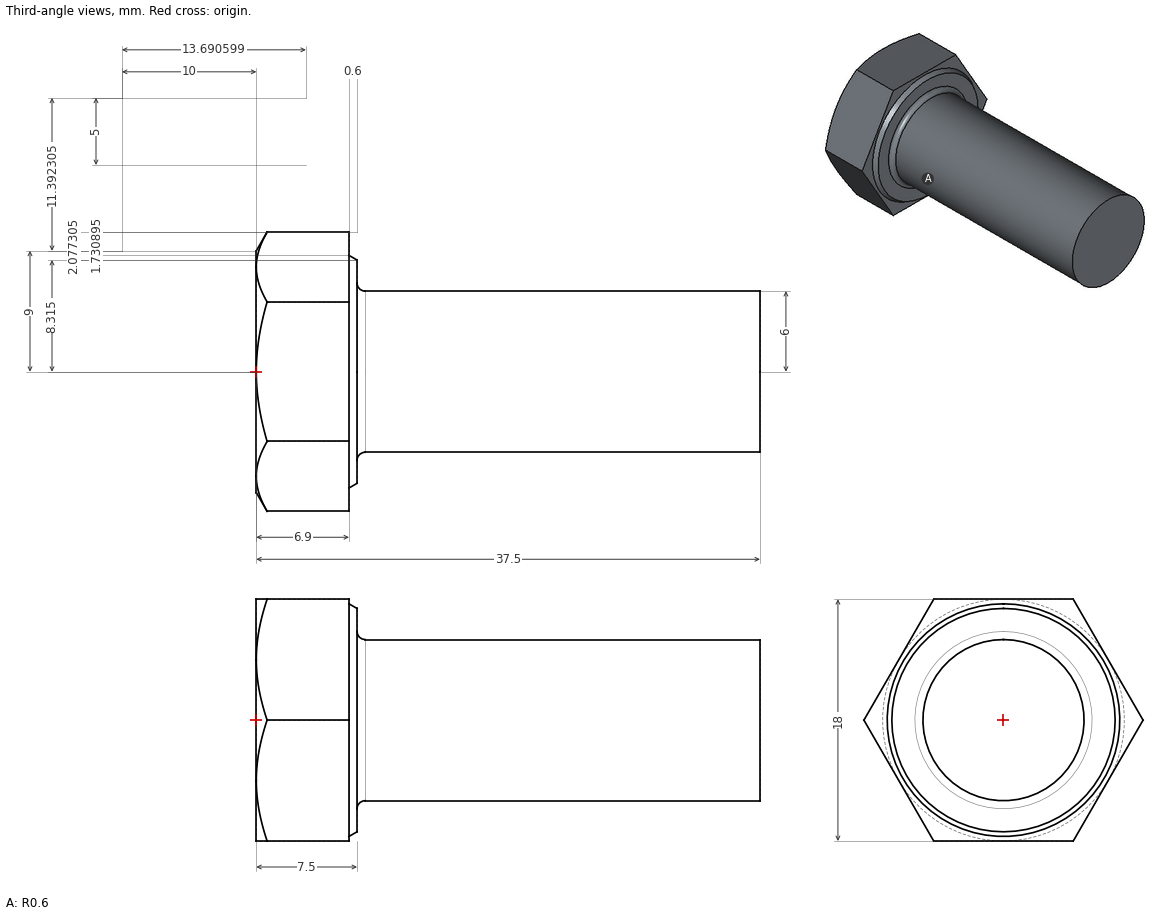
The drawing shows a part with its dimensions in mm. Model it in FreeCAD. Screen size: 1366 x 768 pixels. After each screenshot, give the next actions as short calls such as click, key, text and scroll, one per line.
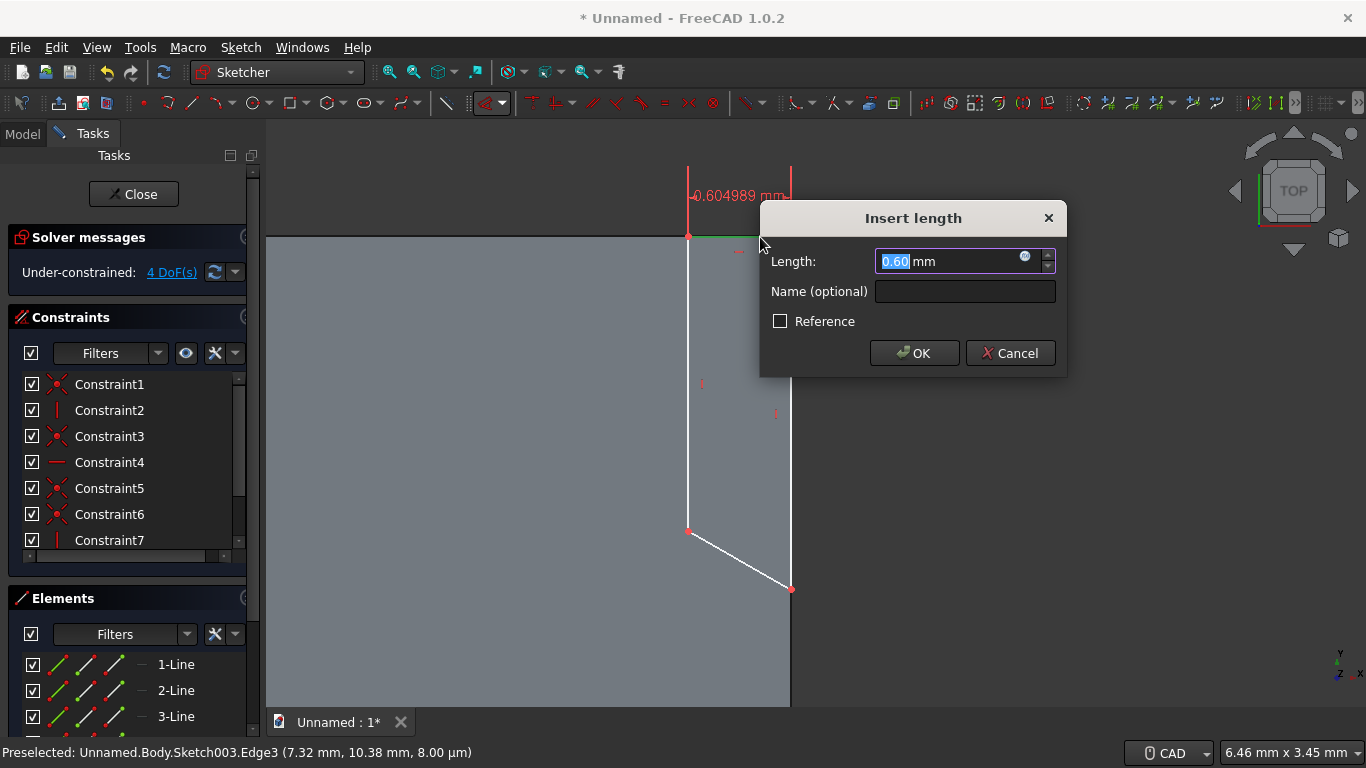
text(0.6)
key(Return)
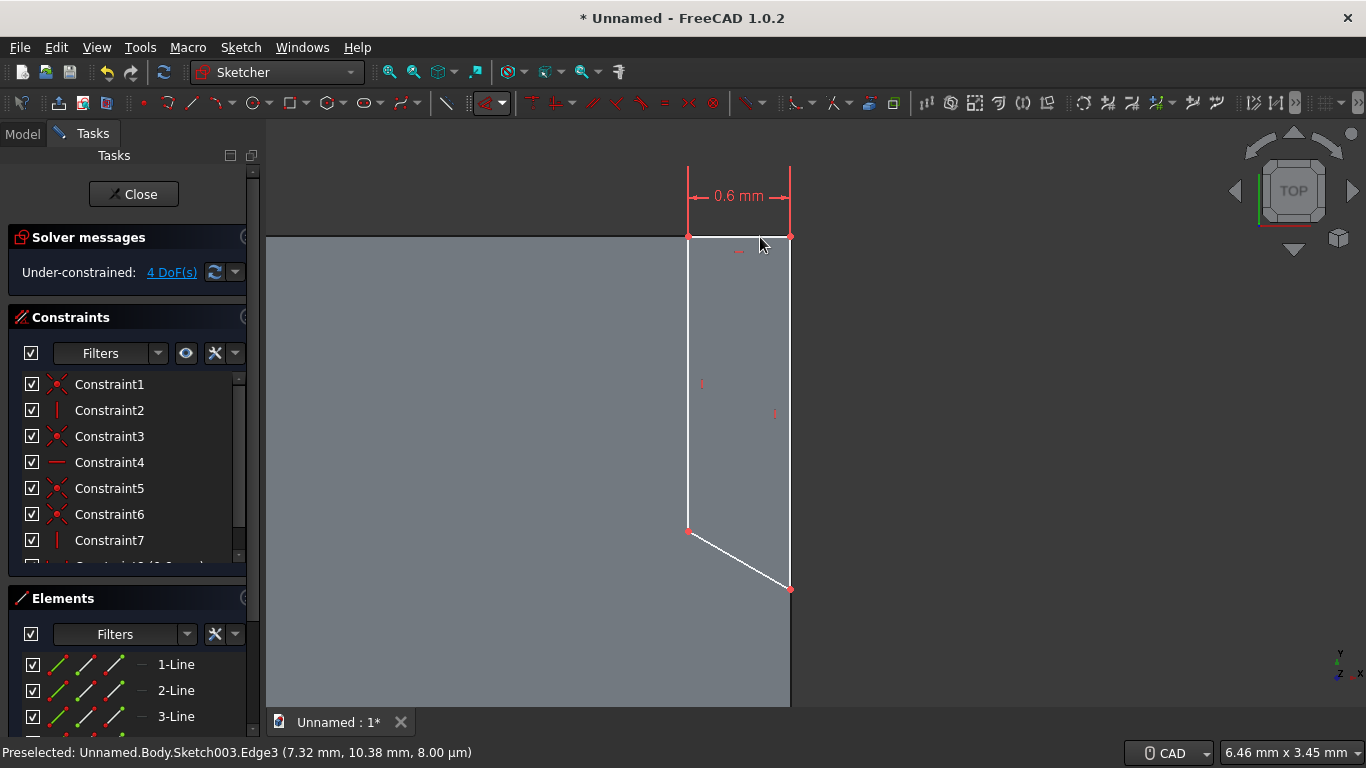
click(688, 531)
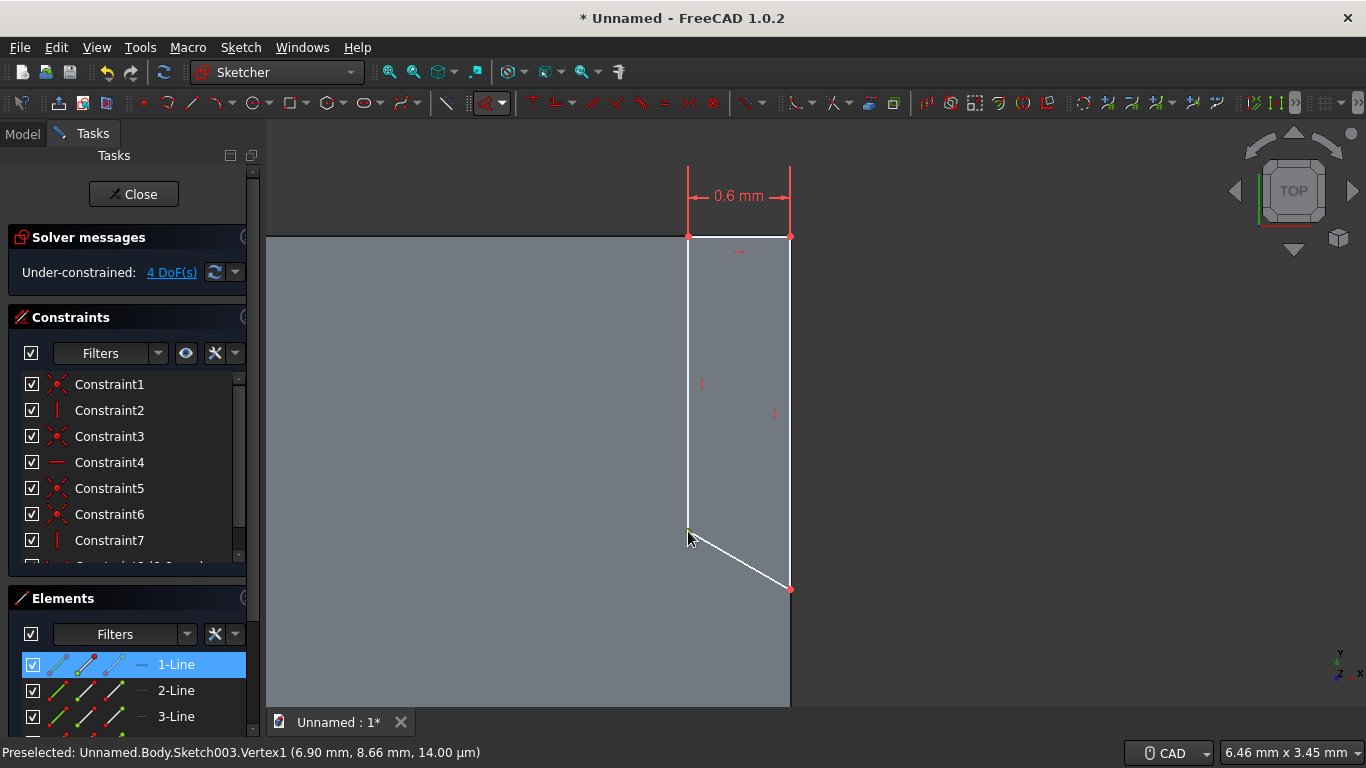
key(l)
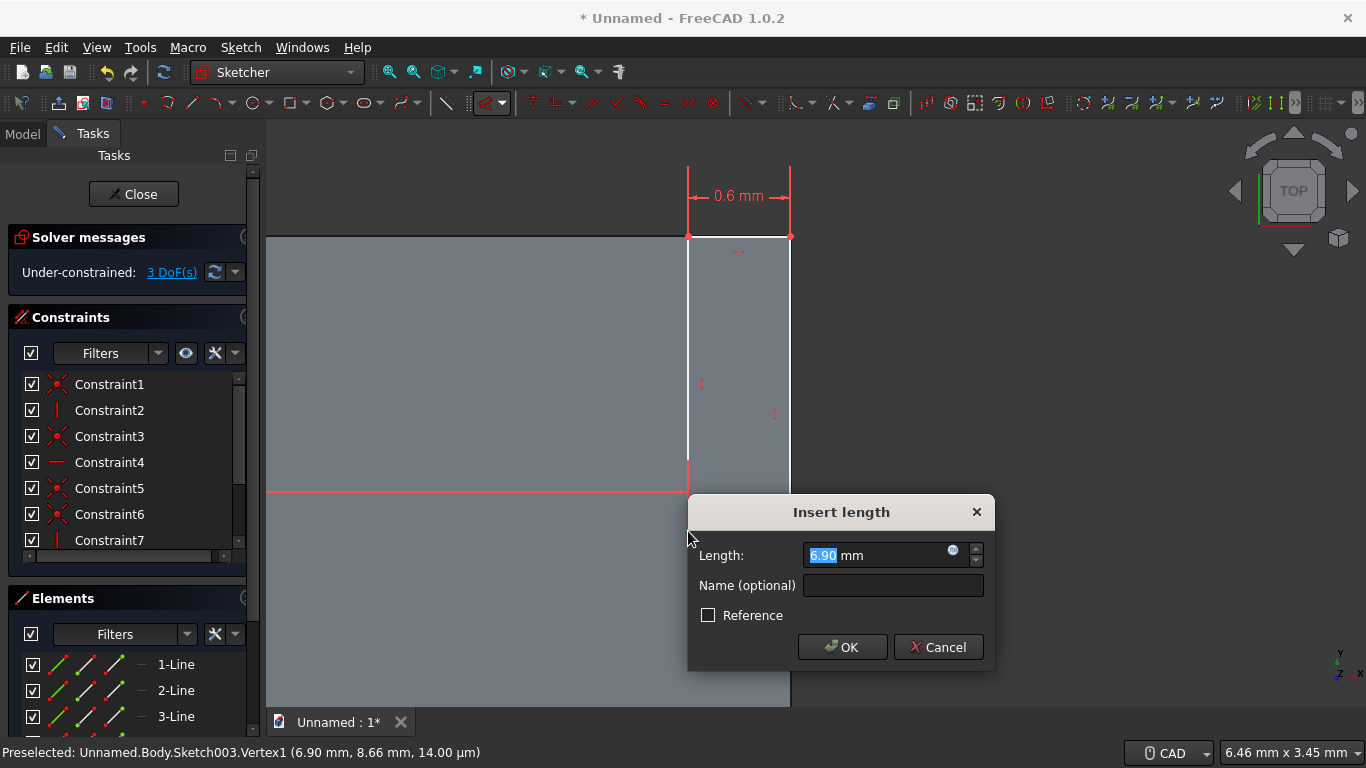
text(6.9)
key(Return)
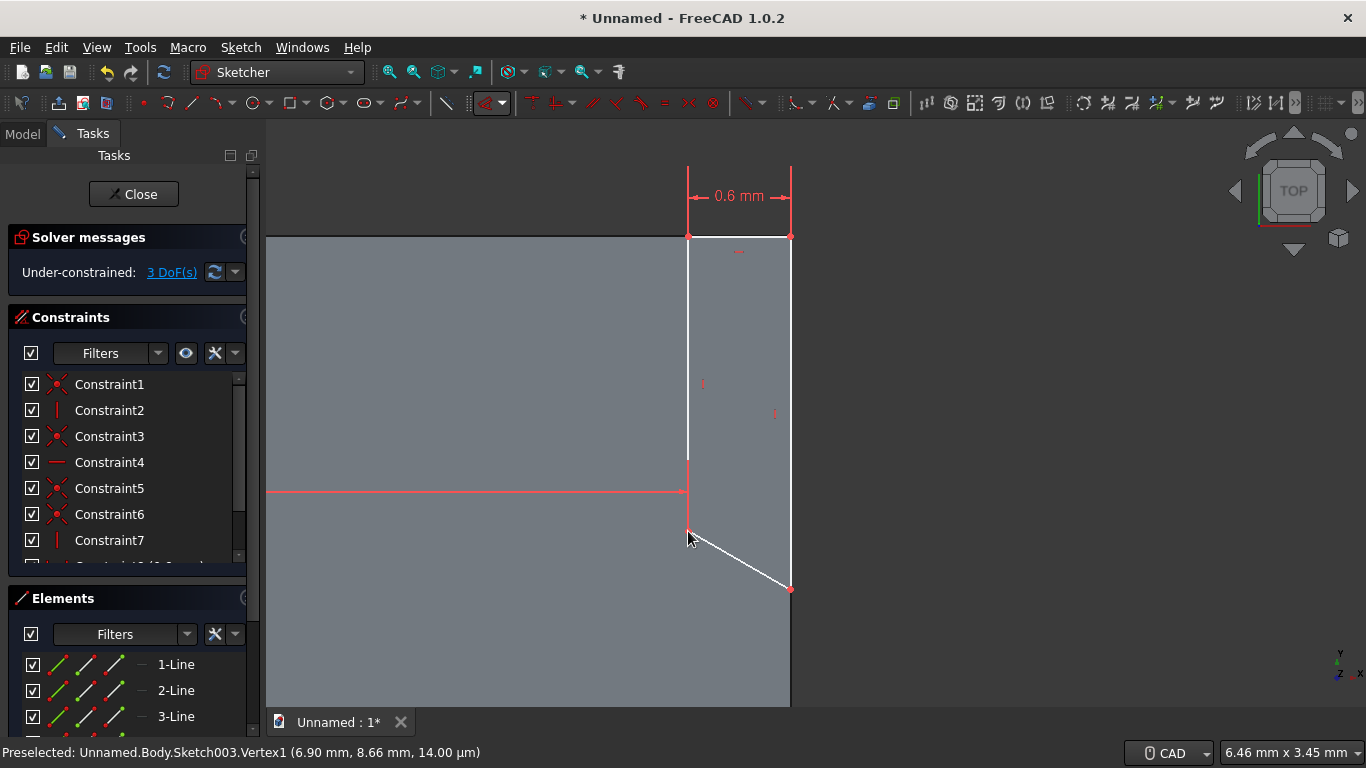
click(791, 590)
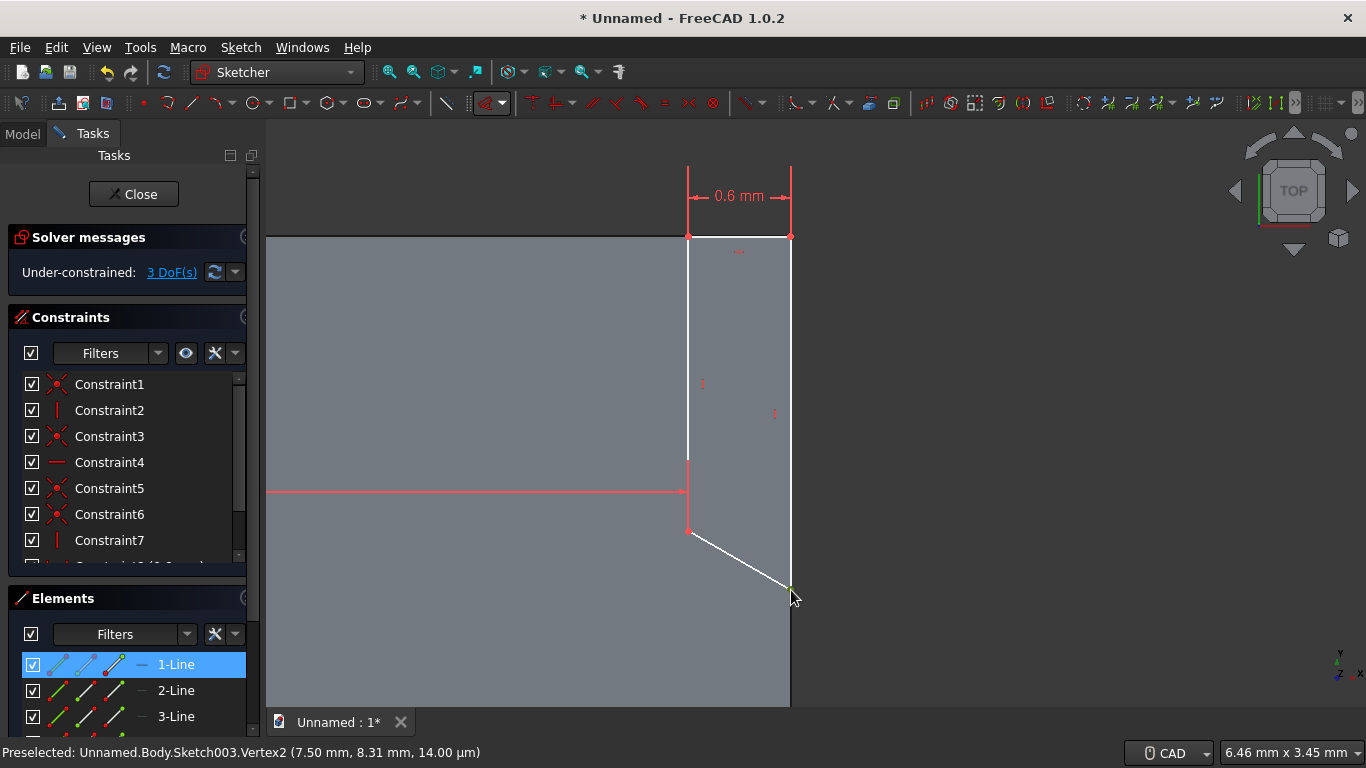
key(i)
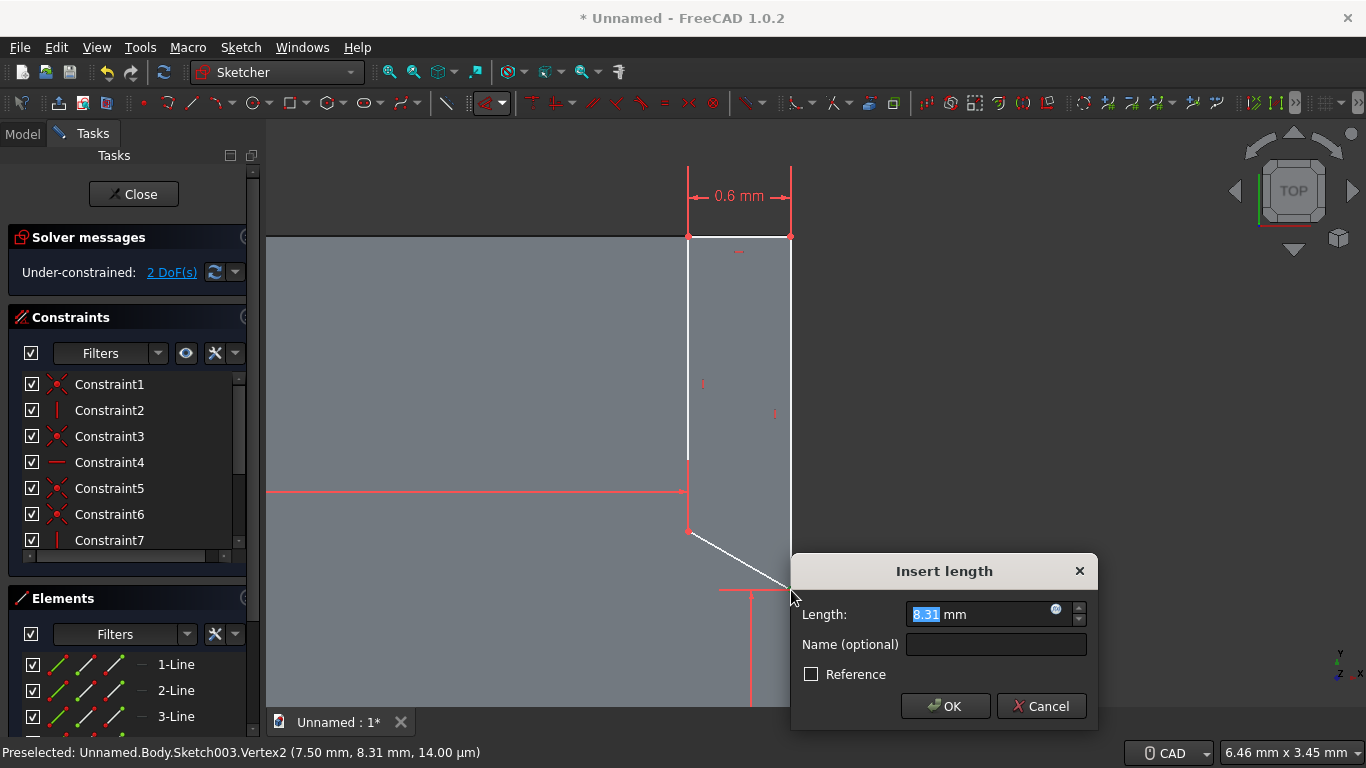
text(8.315)
key(Return)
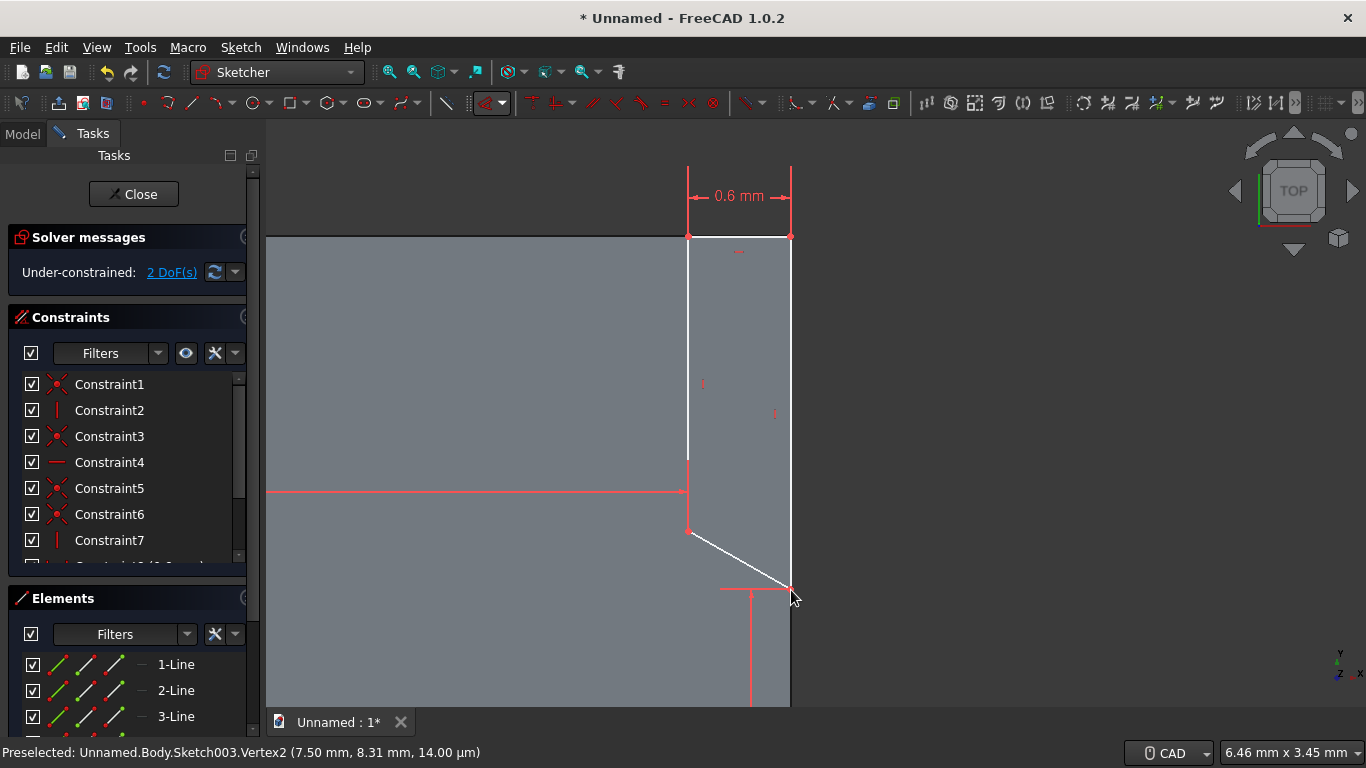
click(791, 484)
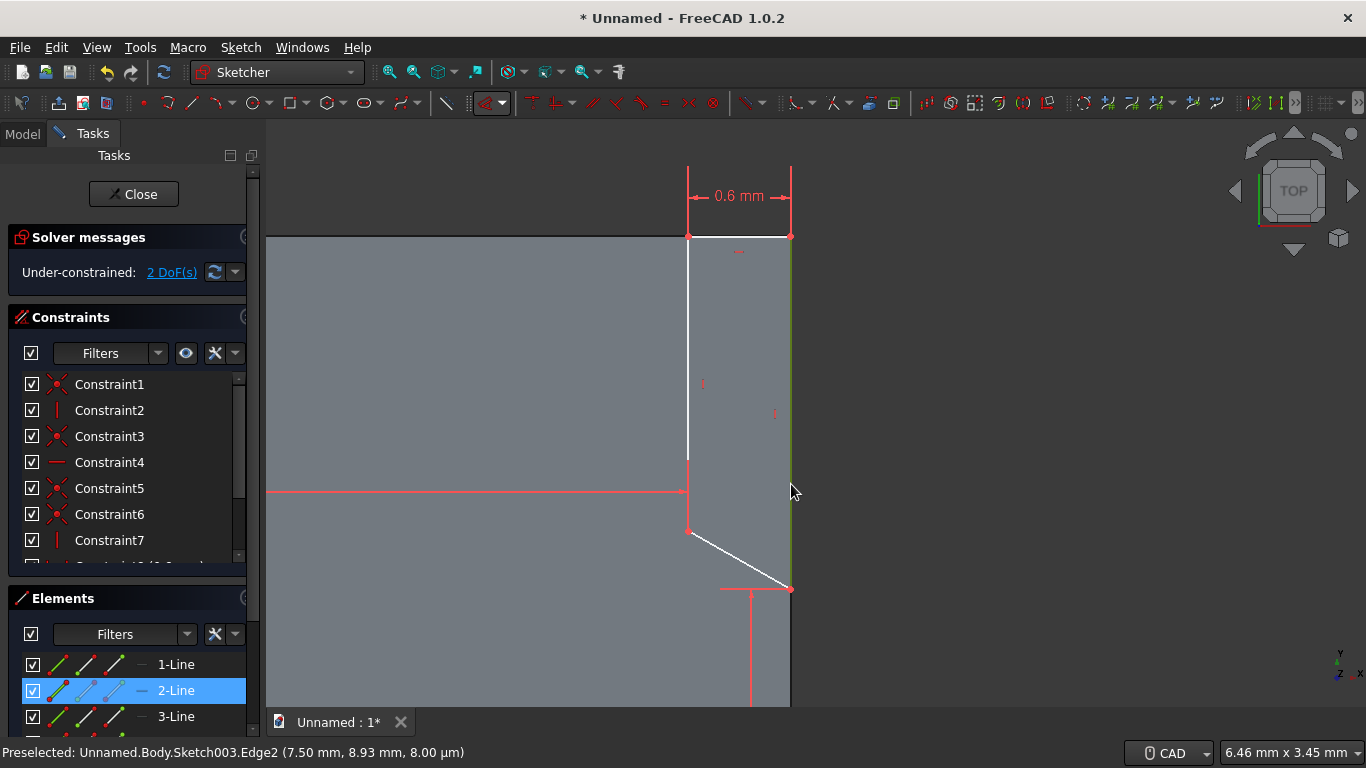
key(i)